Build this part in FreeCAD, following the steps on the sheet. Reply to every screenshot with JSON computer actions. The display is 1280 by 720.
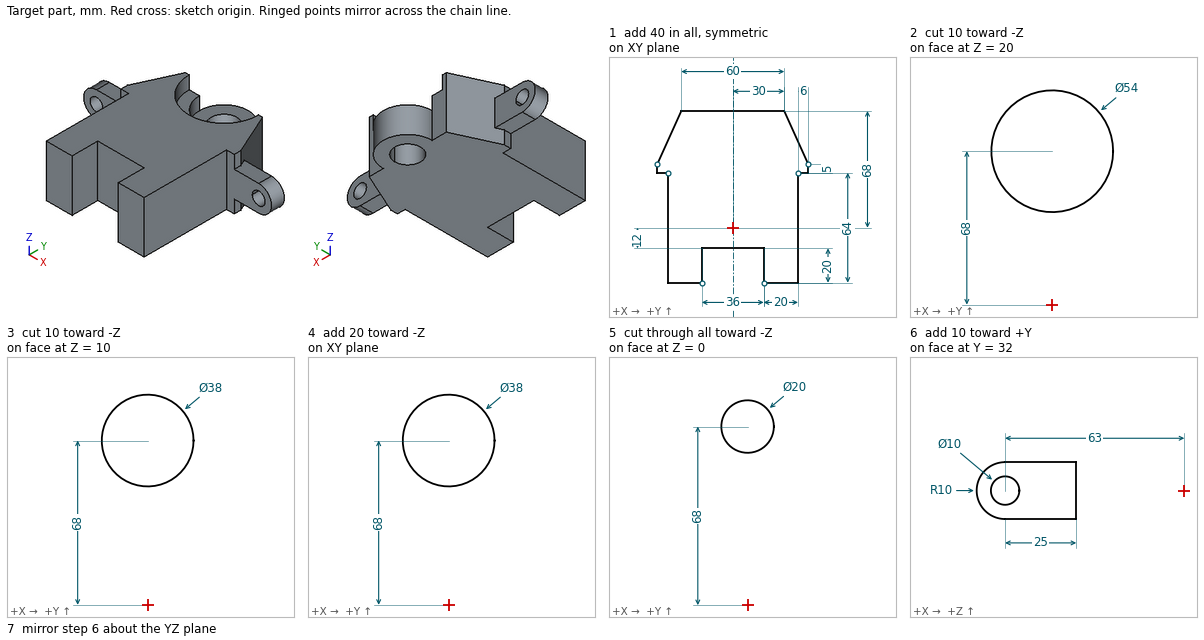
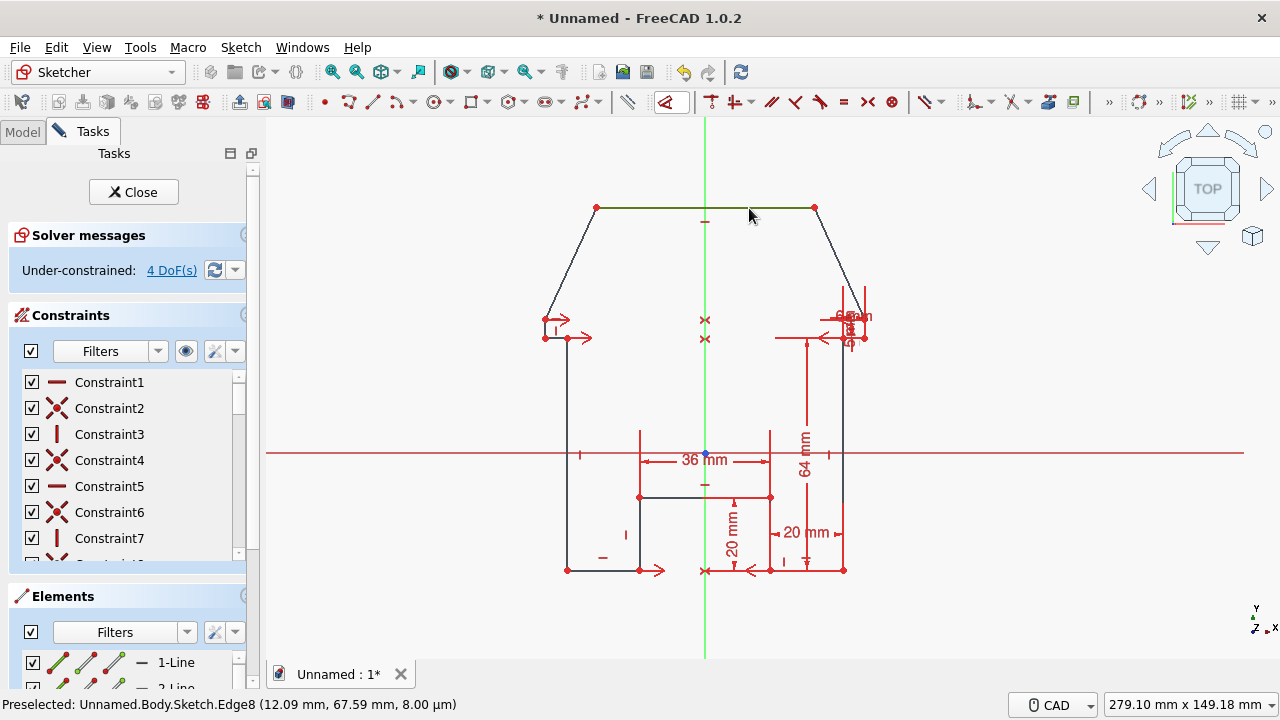
{"action": "left_click", "coordinate": [684, 102]}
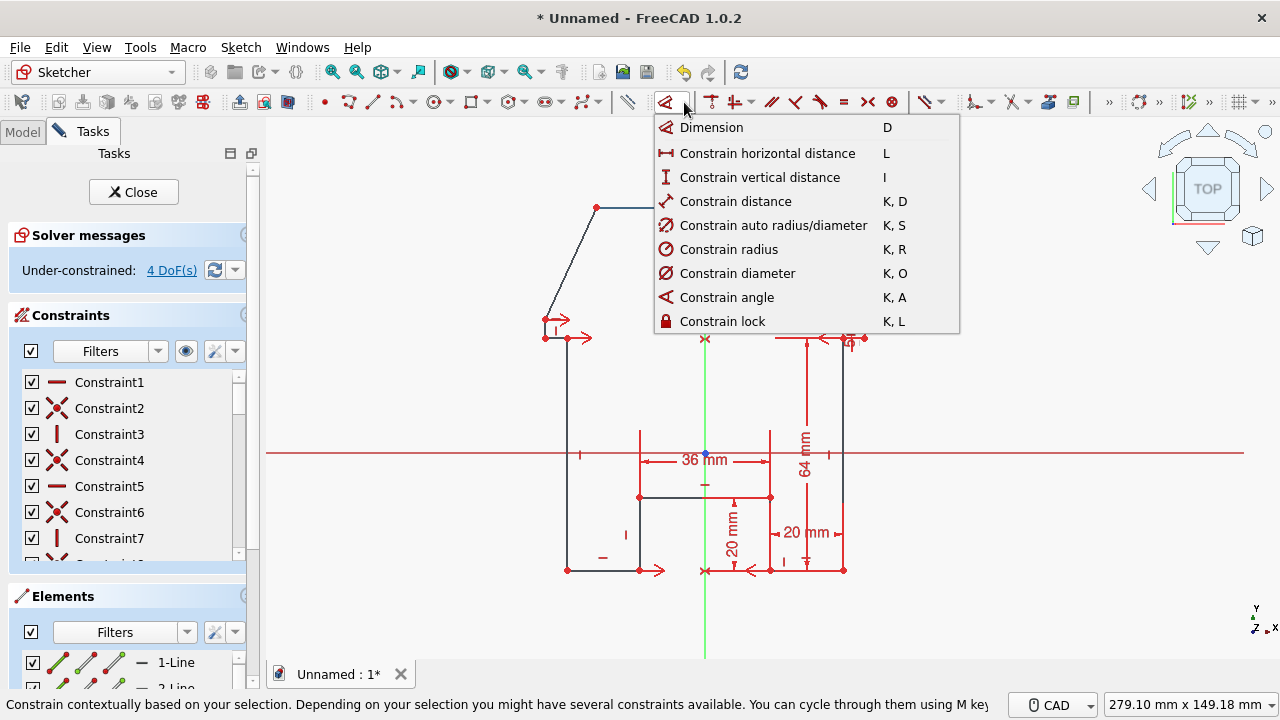
{"action": "left_click", "coordinate": [807, 153]}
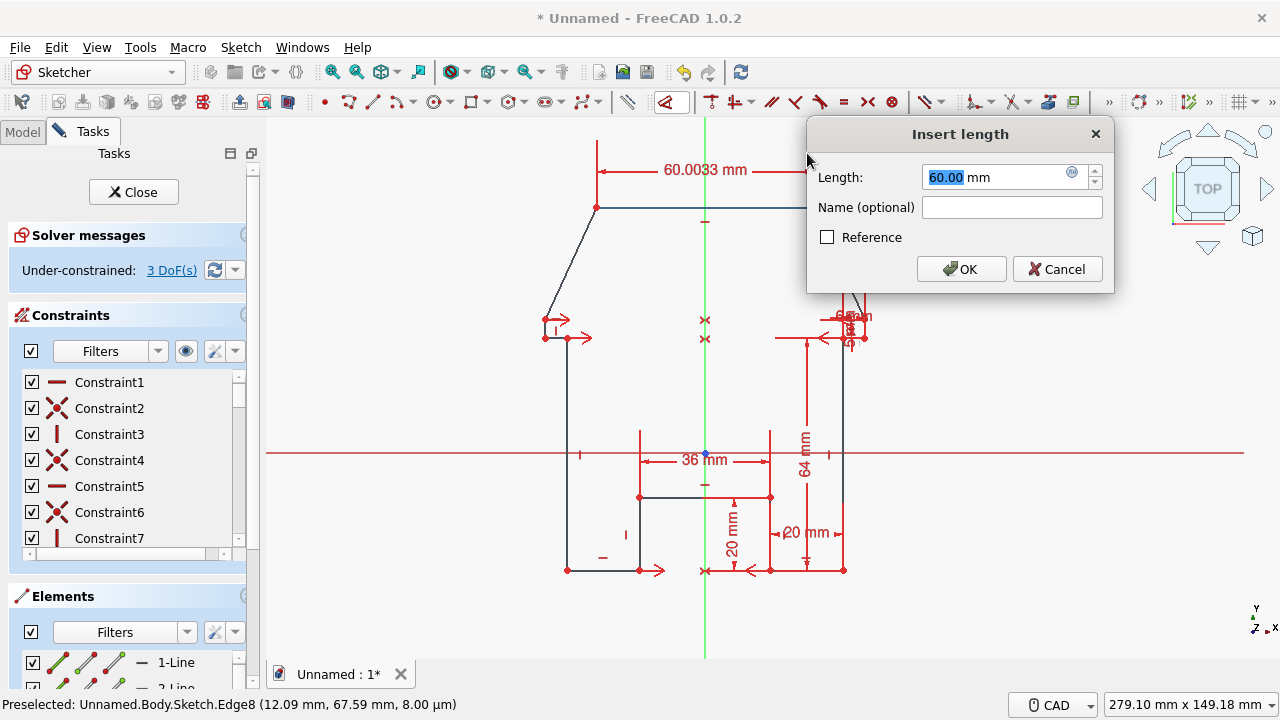
{"action": "type", "text": "60"}
{"action": "key", "text": "Return"}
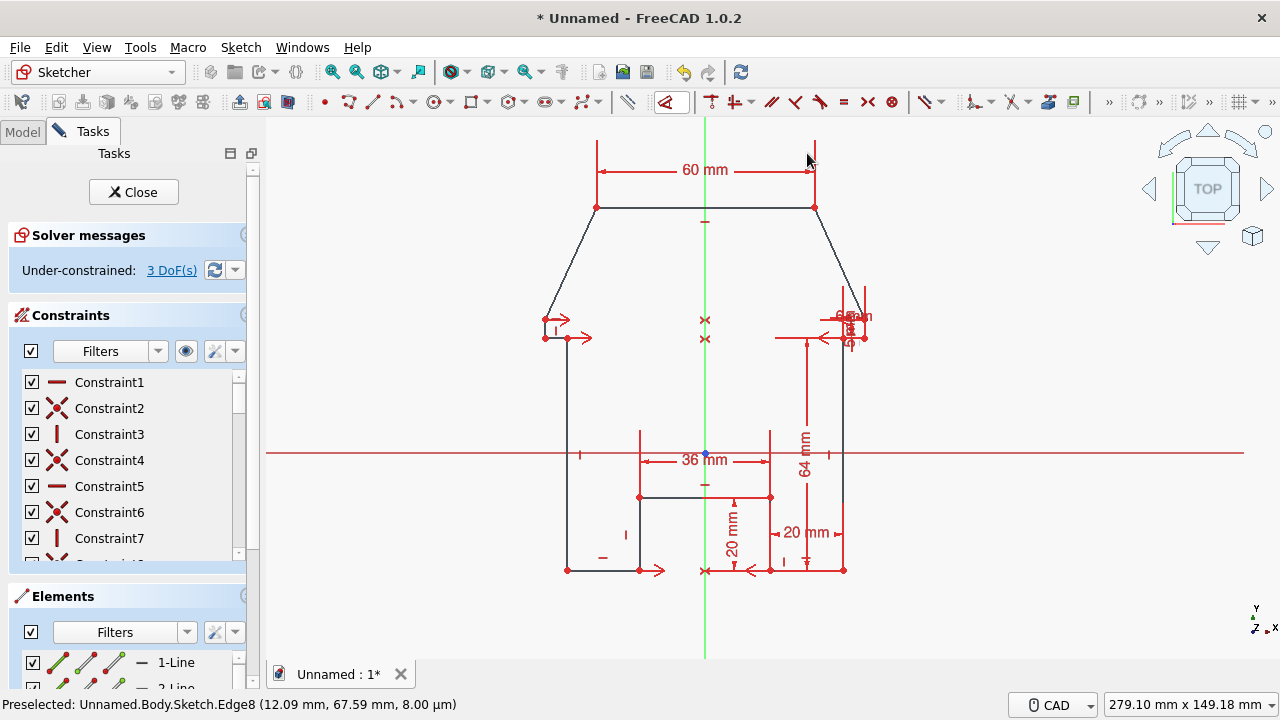
{"action": "left_click", "coordinate": [640, 498]}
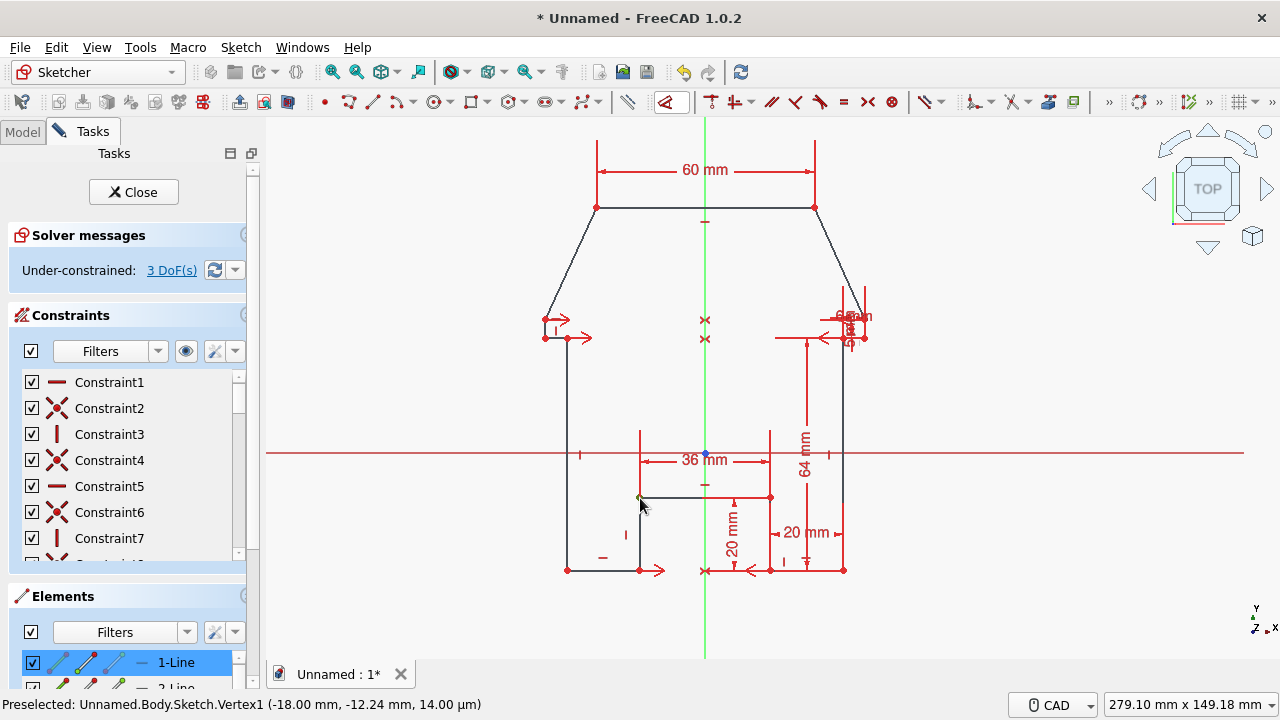
{"action": "left_click", "coordinate": [684, 102]}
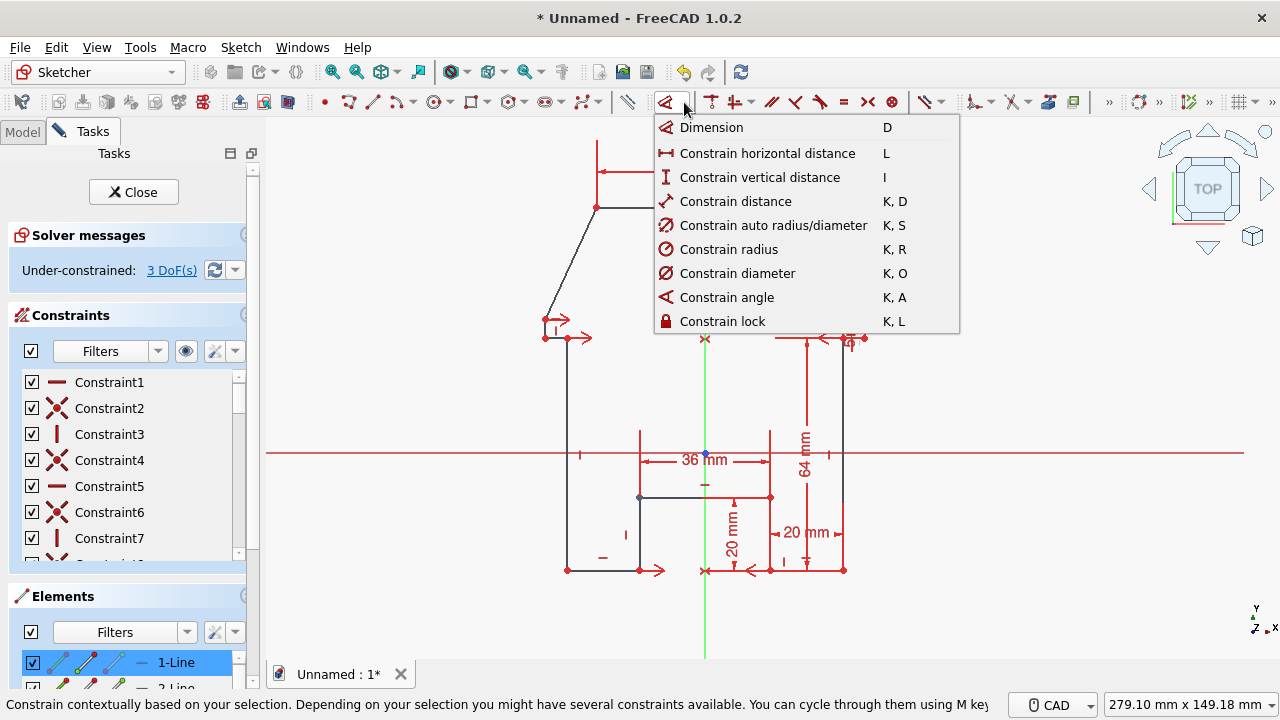
{"action": "left_click", "coordinate": [807, 177]}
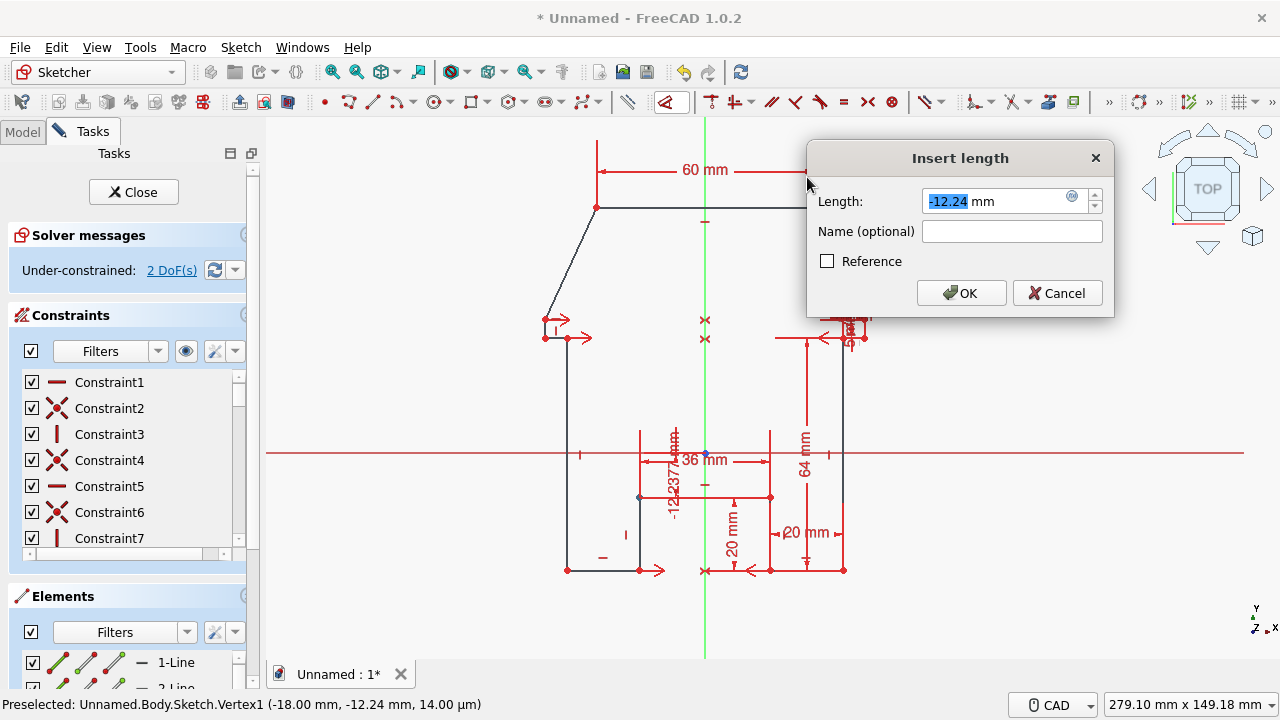
{"action": "type", "text": "-12"}
{"action": "key", "text": "Return"}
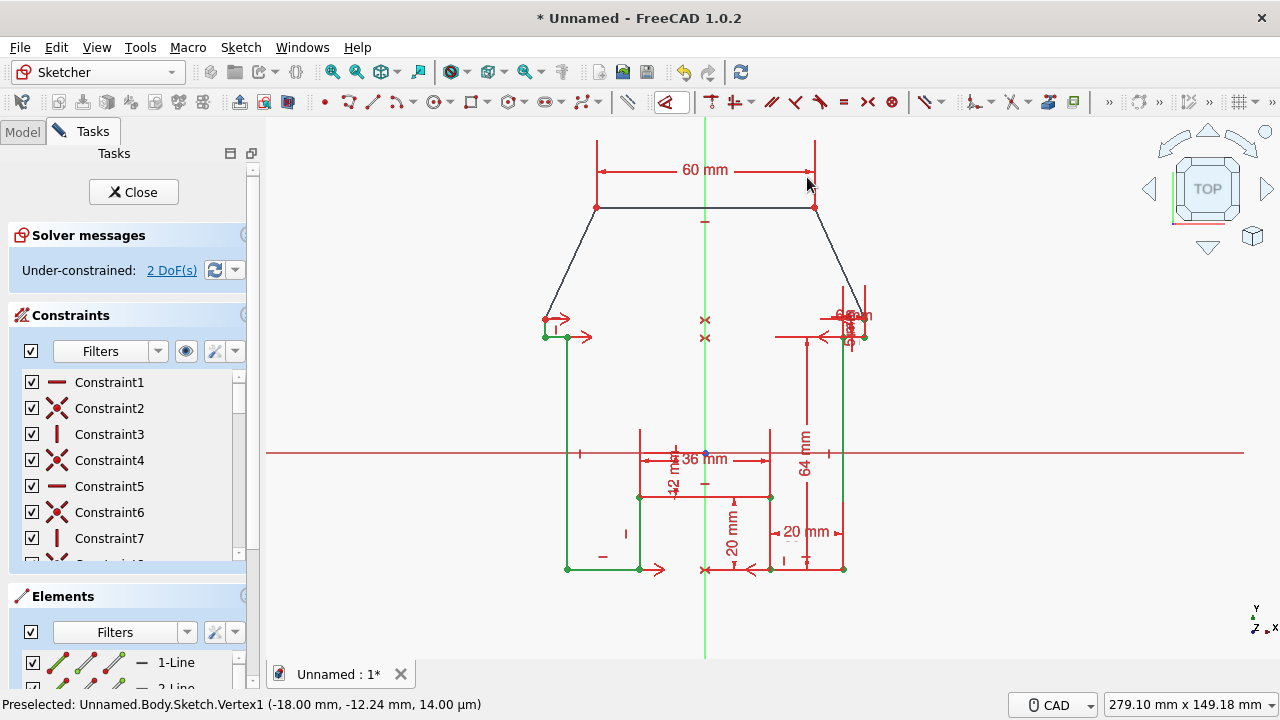
{"action": "left_click", "coordinate": [815, 208]}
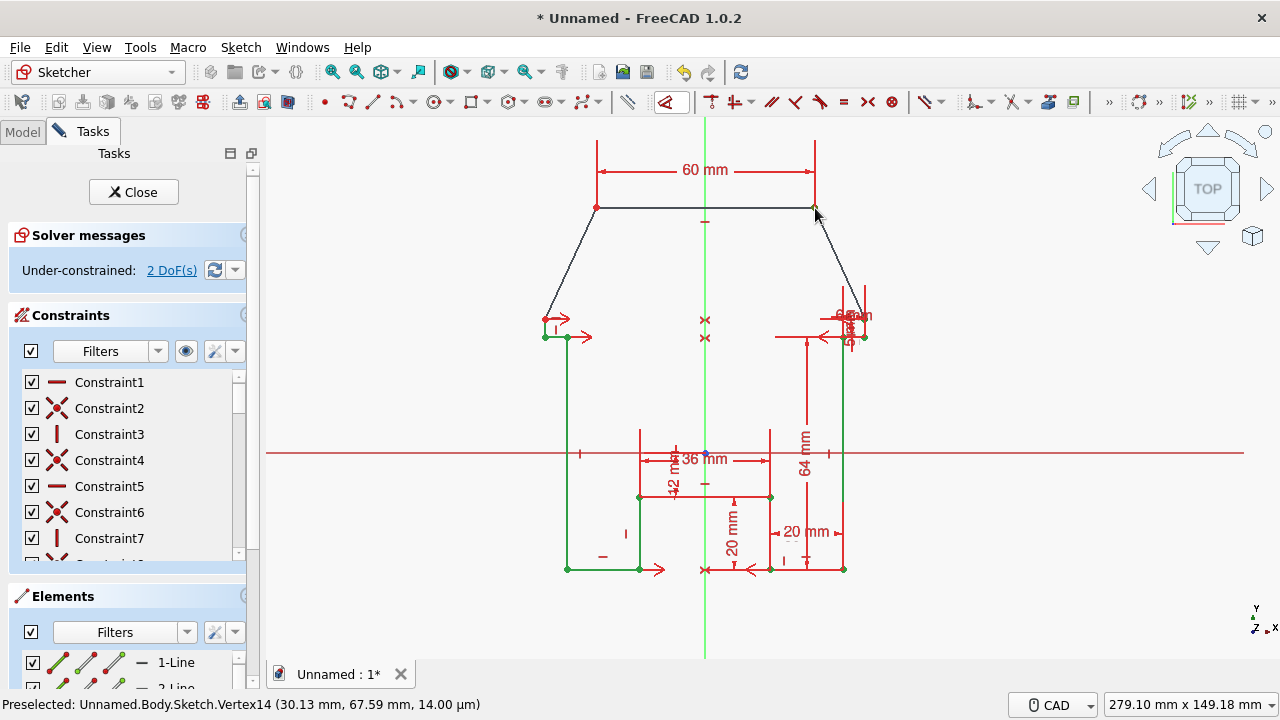
{"action": "left_click", "coordinate": [684, 102]}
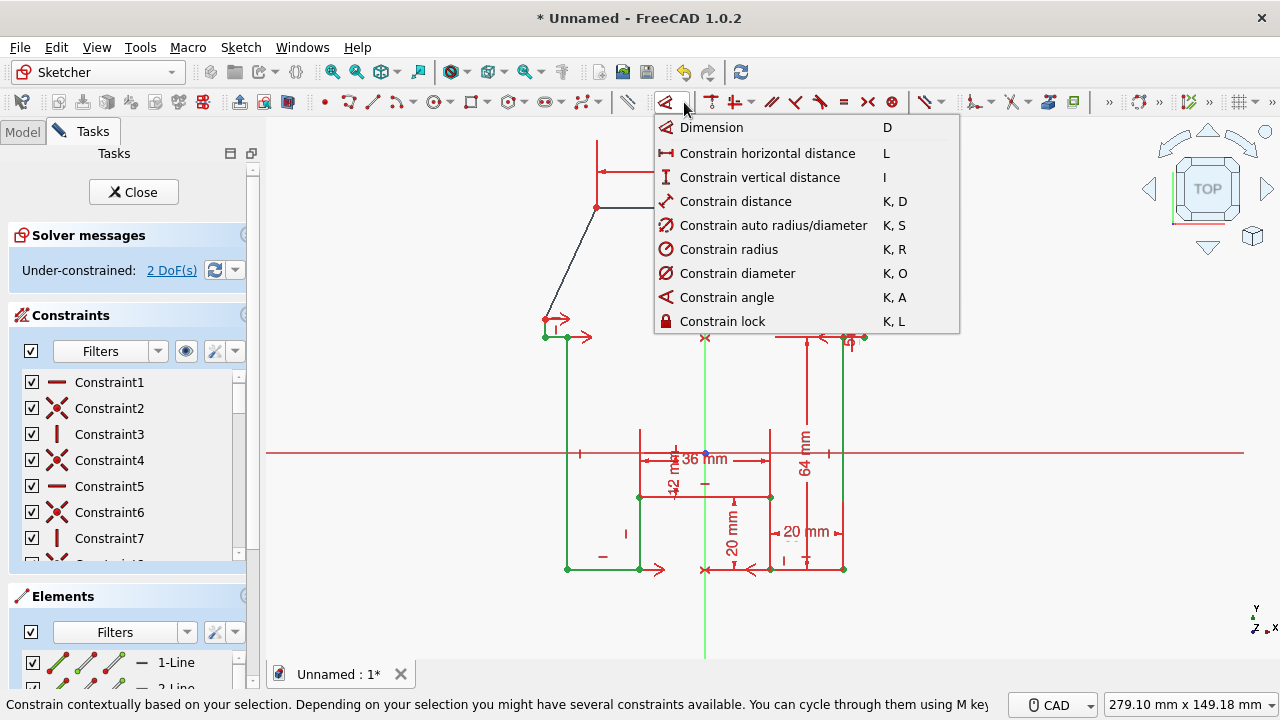
{"action": "left_click", "coordinate": [807, 153]}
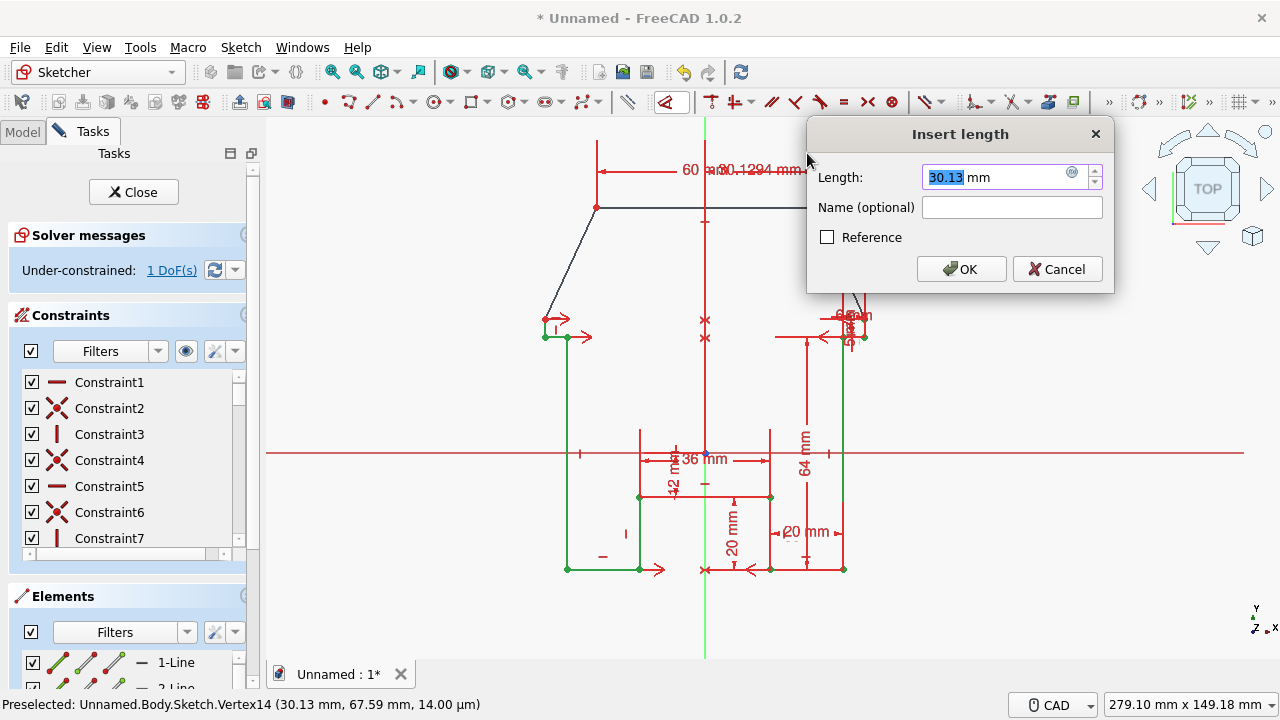
{"action": "type", "text": "30"}
{"action": "key", "text": "Return"}